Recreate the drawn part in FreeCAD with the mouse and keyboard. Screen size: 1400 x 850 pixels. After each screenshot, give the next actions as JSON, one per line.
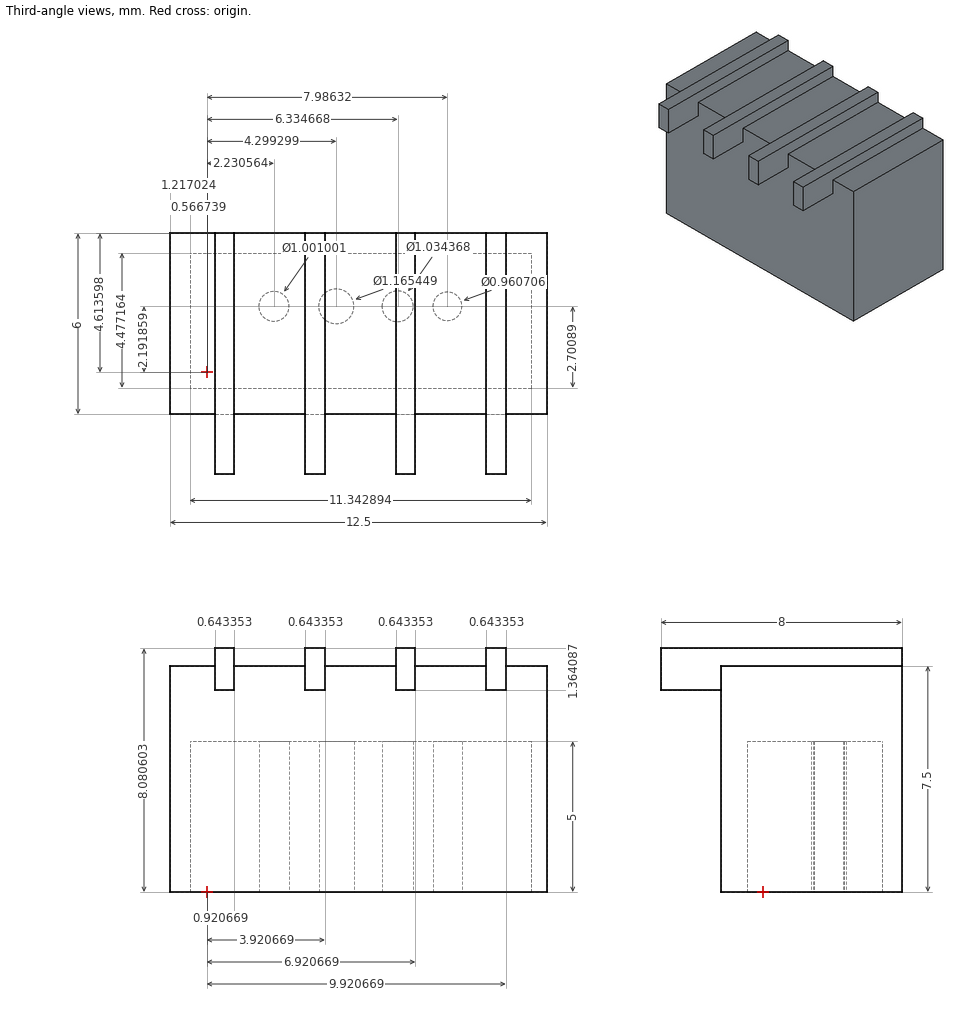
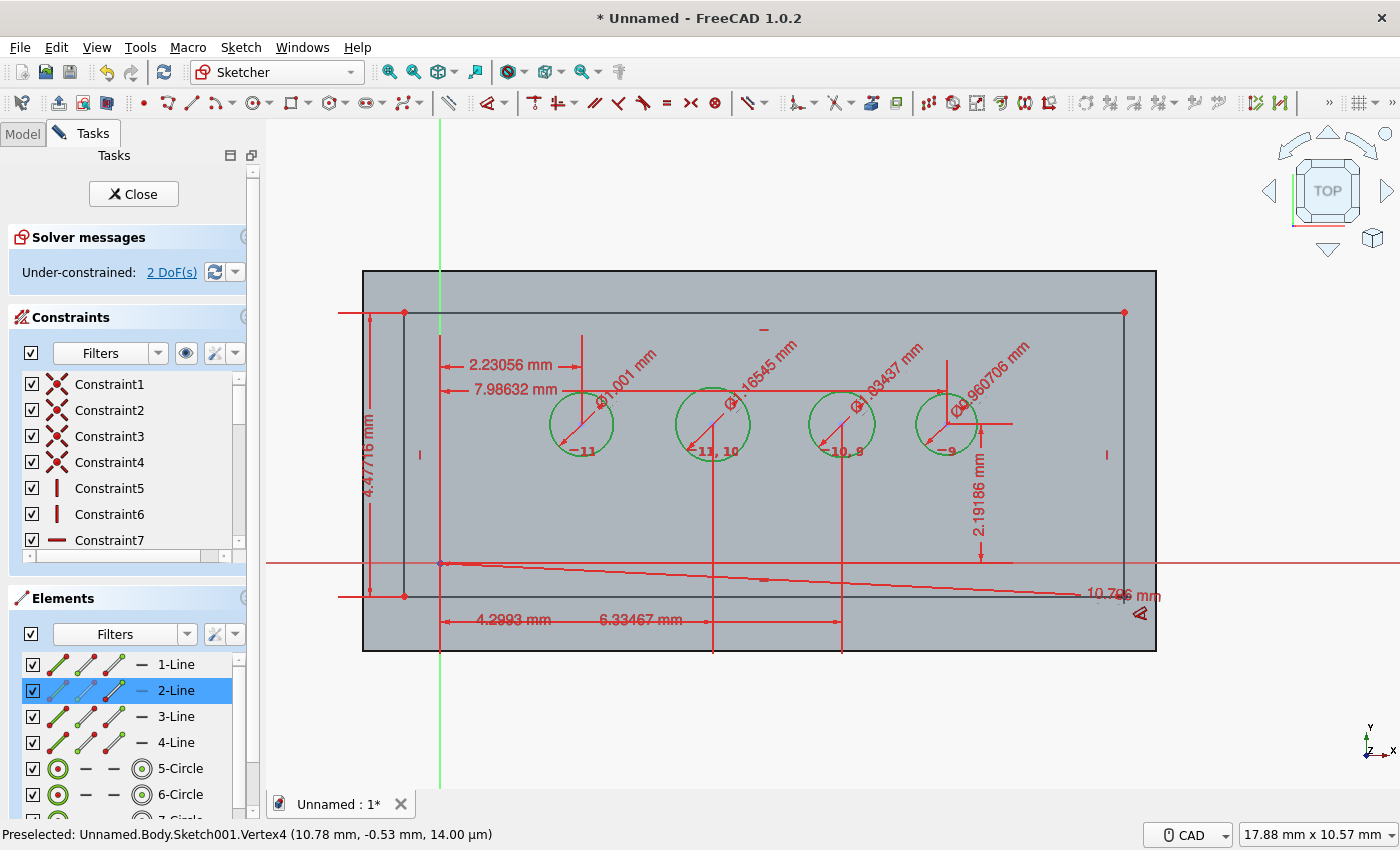
{"action": "left_click", "coordinate": [947, 424]}
{"action": "left_click", "coordinate": [1158, 511]}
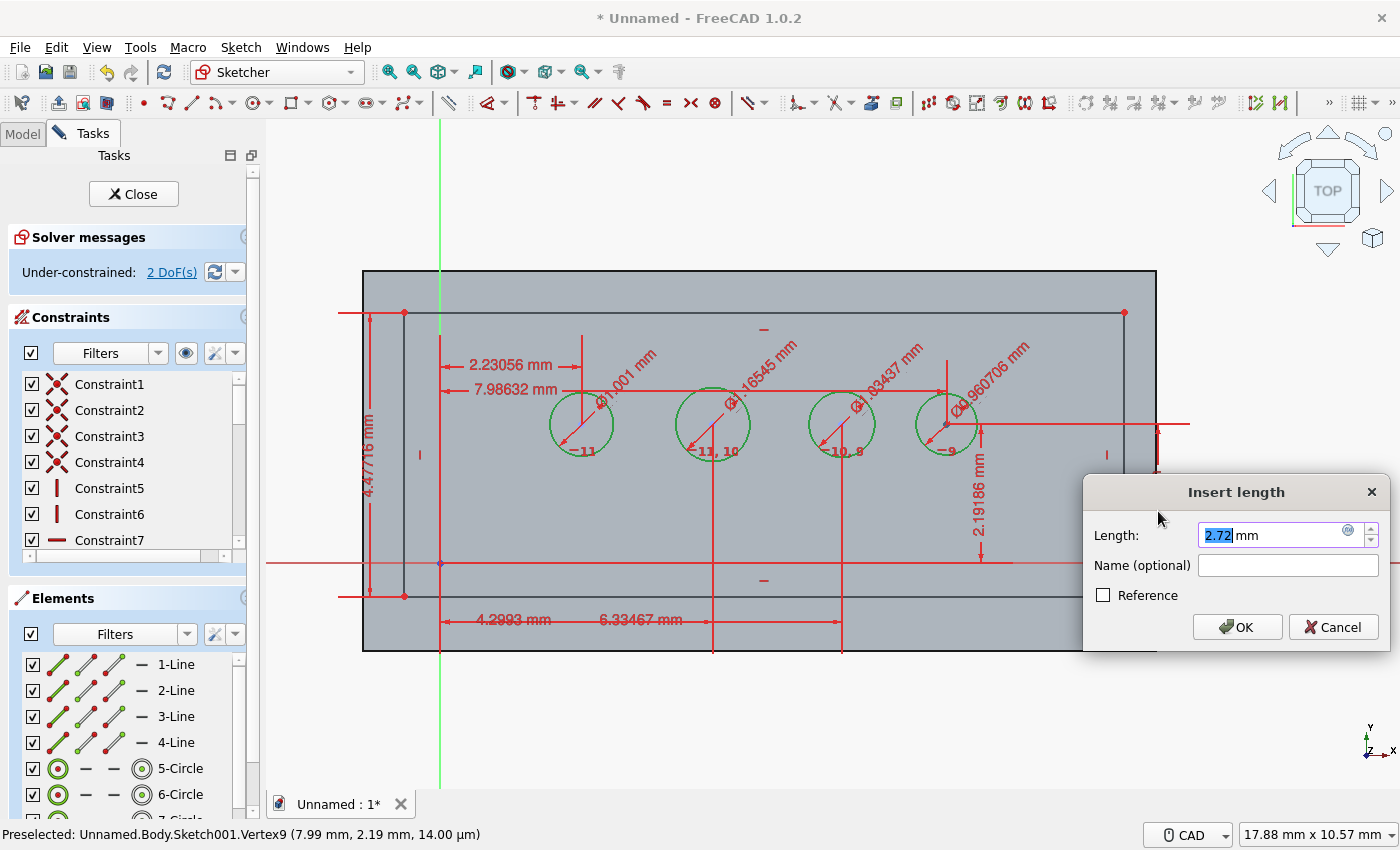
{"action": "type", "text": "2.70089"}
{"action": "key", "text": "Return"}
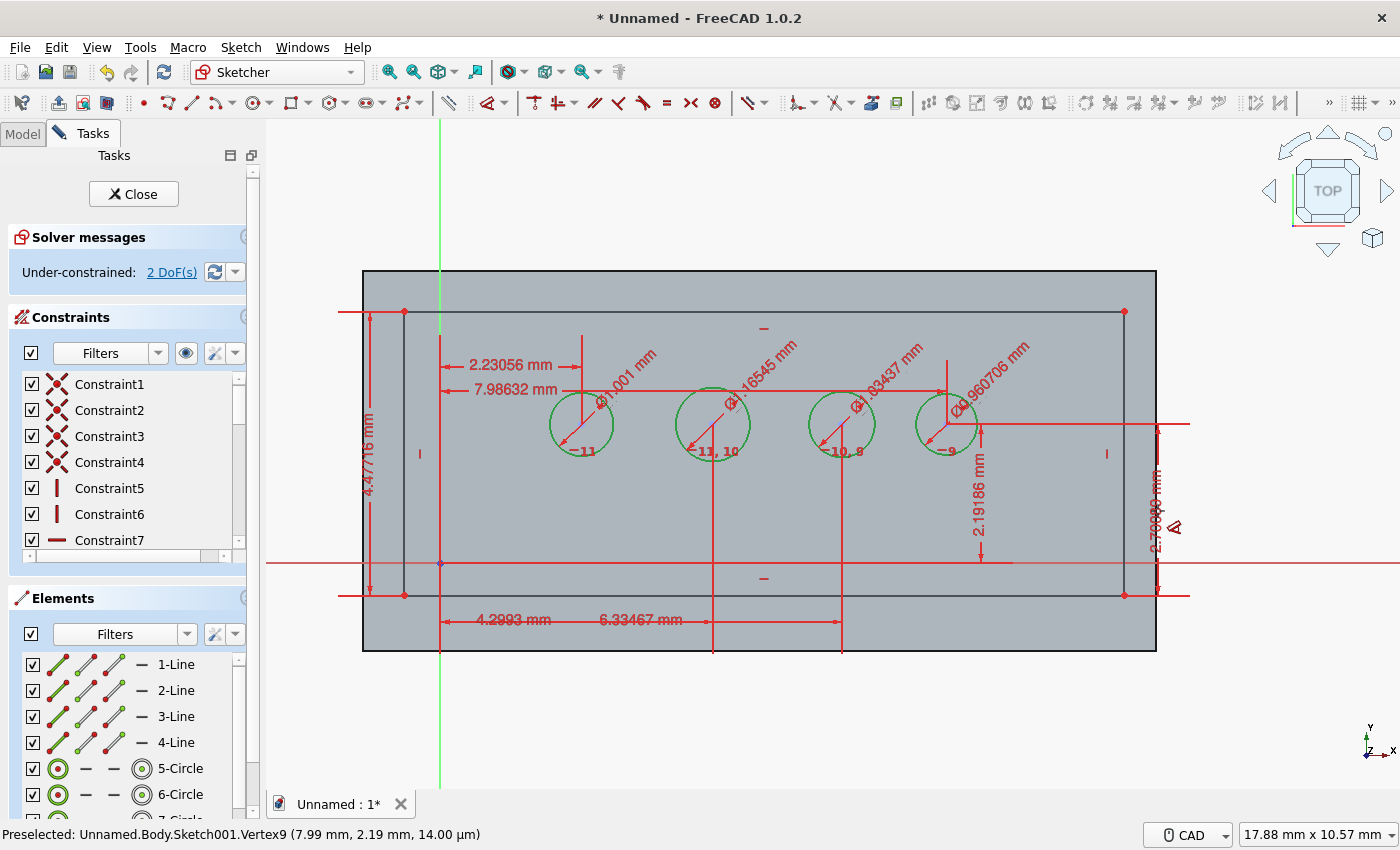
{"action": "left_click", "coordinate": [620, 596]}
{"action": "left_click", "coordinate": [764, 630]}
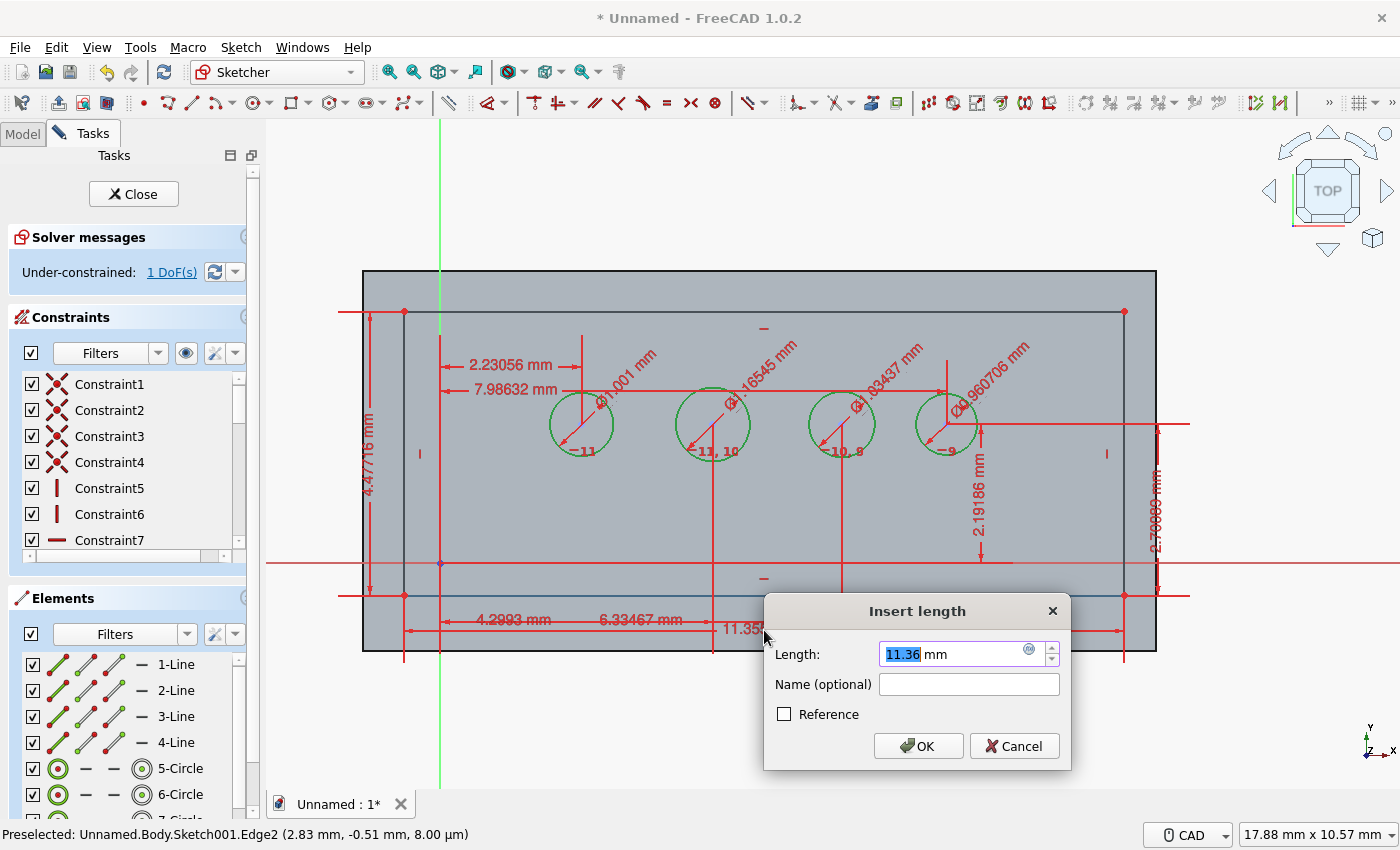
{"action": "type", "text": "11.342894"}
{"action": "key", "text": "Return"}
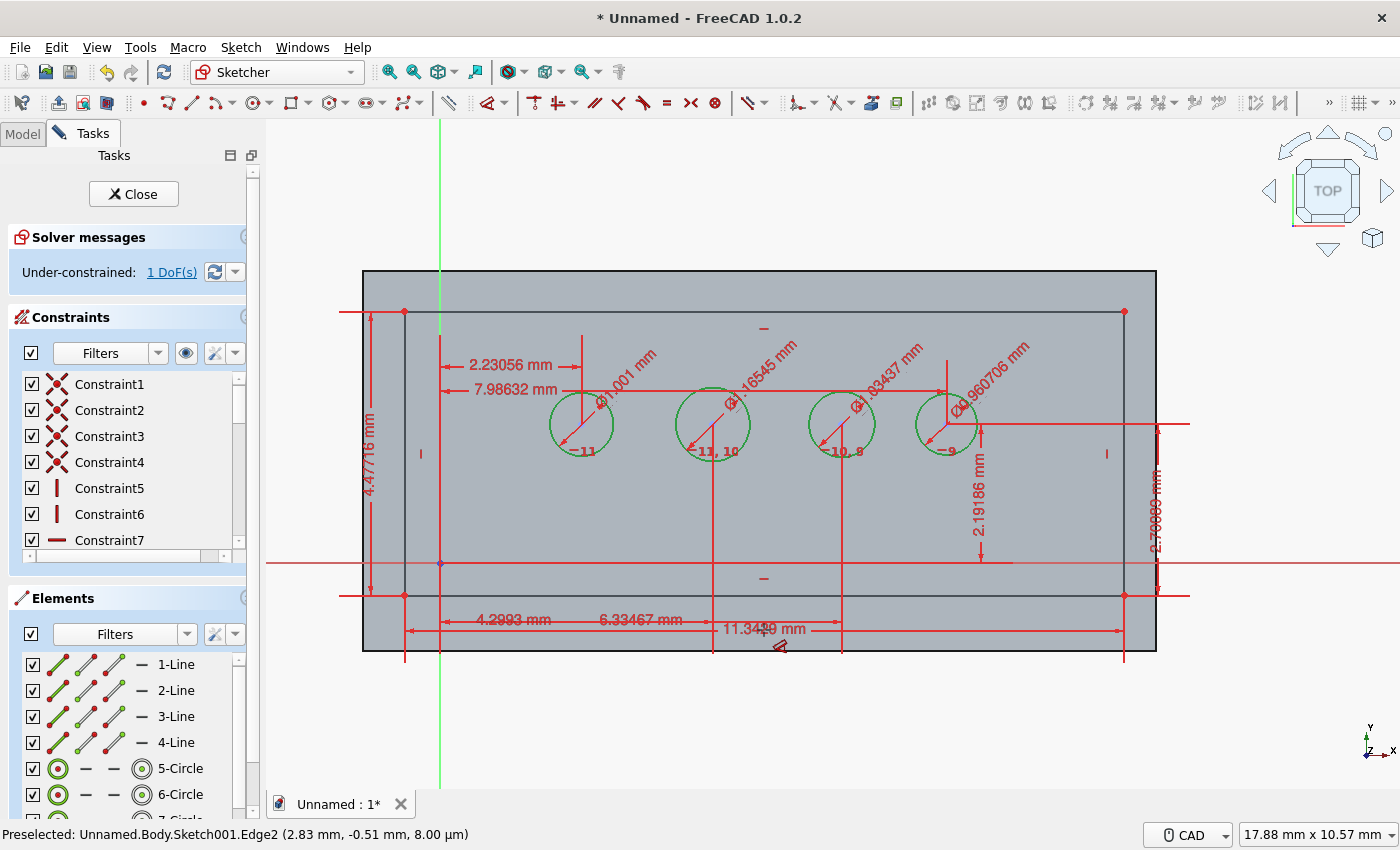
{"action": "left_click", "coordinate": [405, 312]}
{"action": "left_click", "coordinate": [423, 278]}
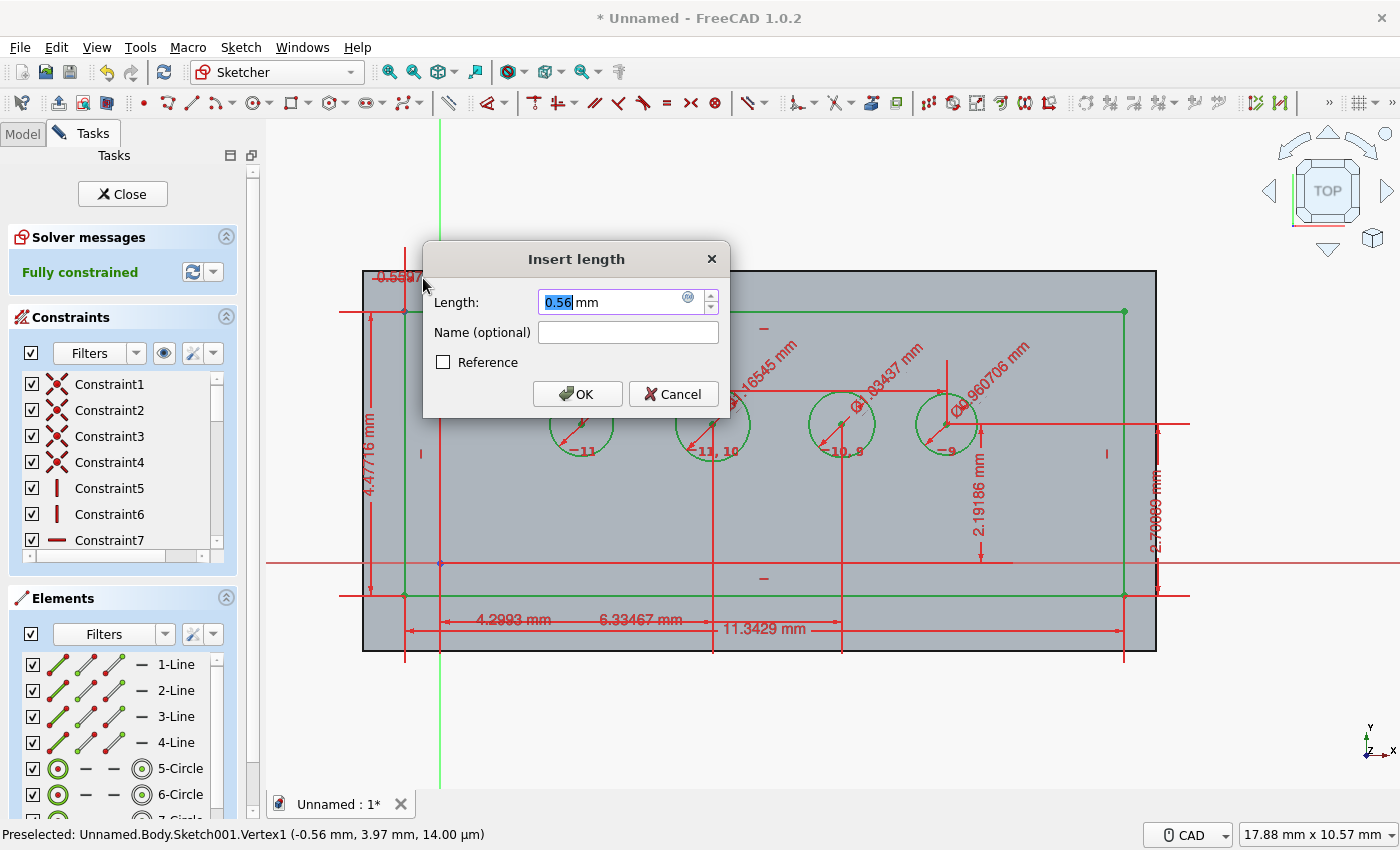
{"action": "type", "text": "0.566739"}
{"action": "key", "text": "Return"}
{"action": "key", "text": "Escape"}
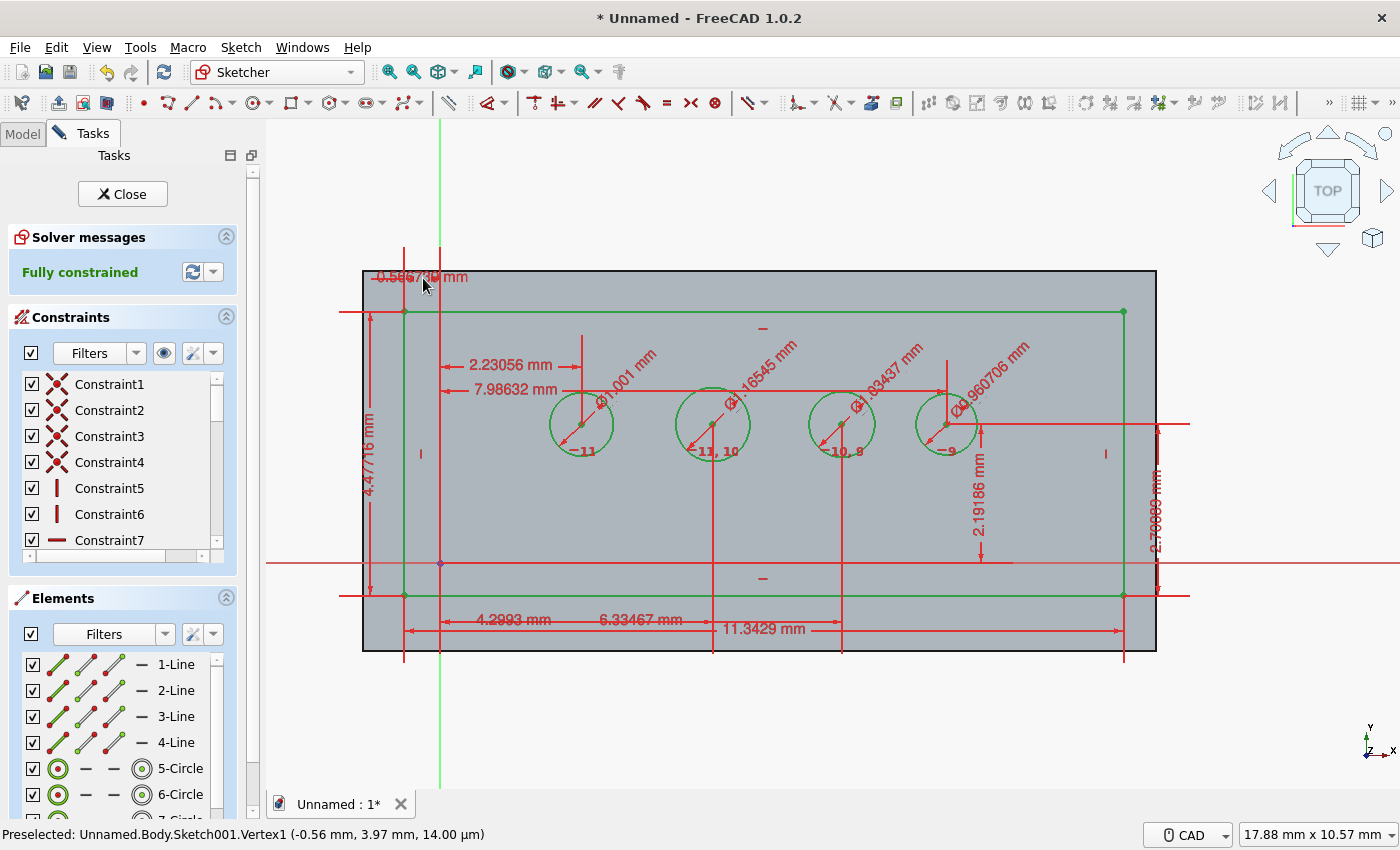
{"action": "left_click", "coordinate": [123, 194]}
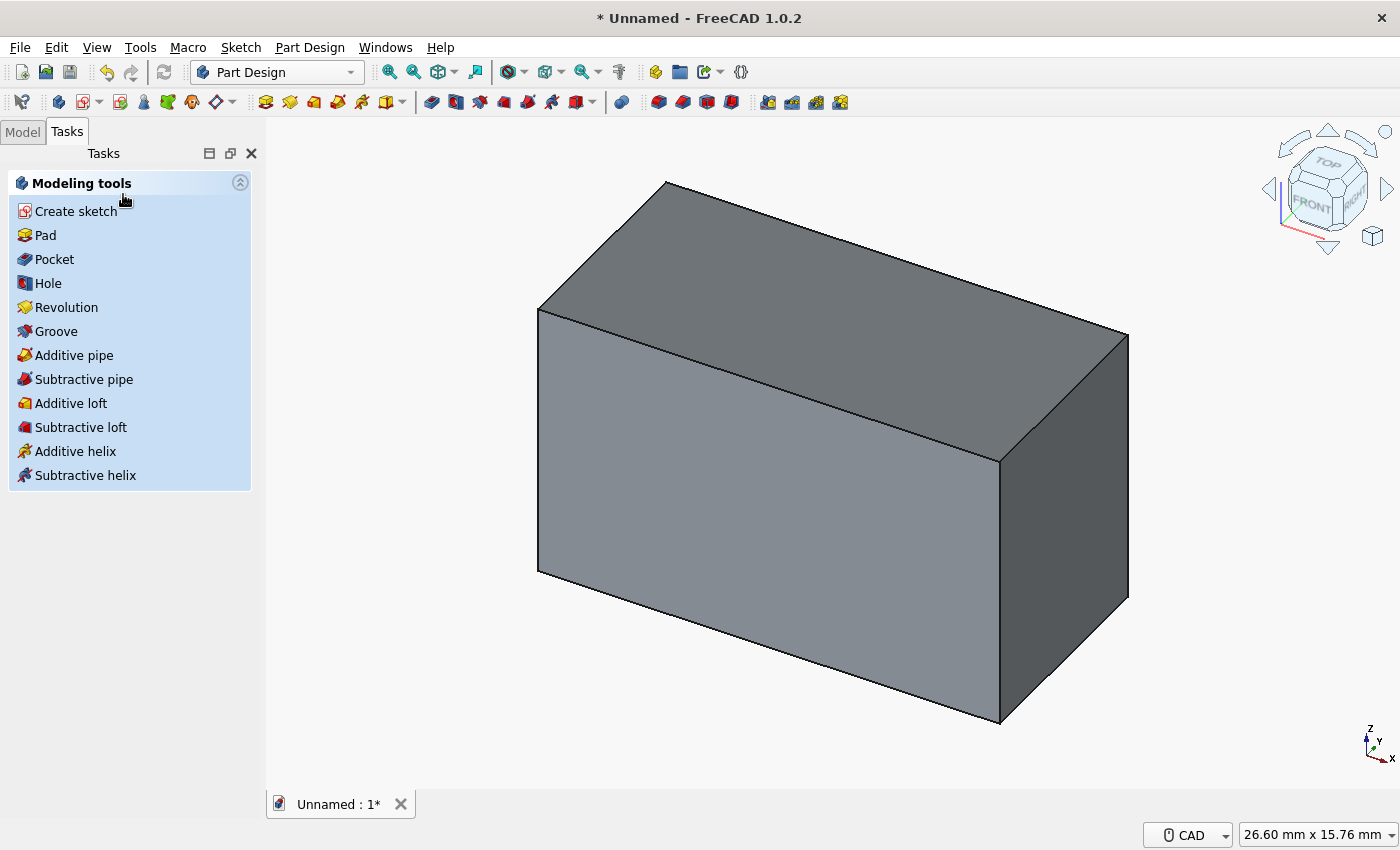
{"action": "left_click", "coordinate": [432, 102]}